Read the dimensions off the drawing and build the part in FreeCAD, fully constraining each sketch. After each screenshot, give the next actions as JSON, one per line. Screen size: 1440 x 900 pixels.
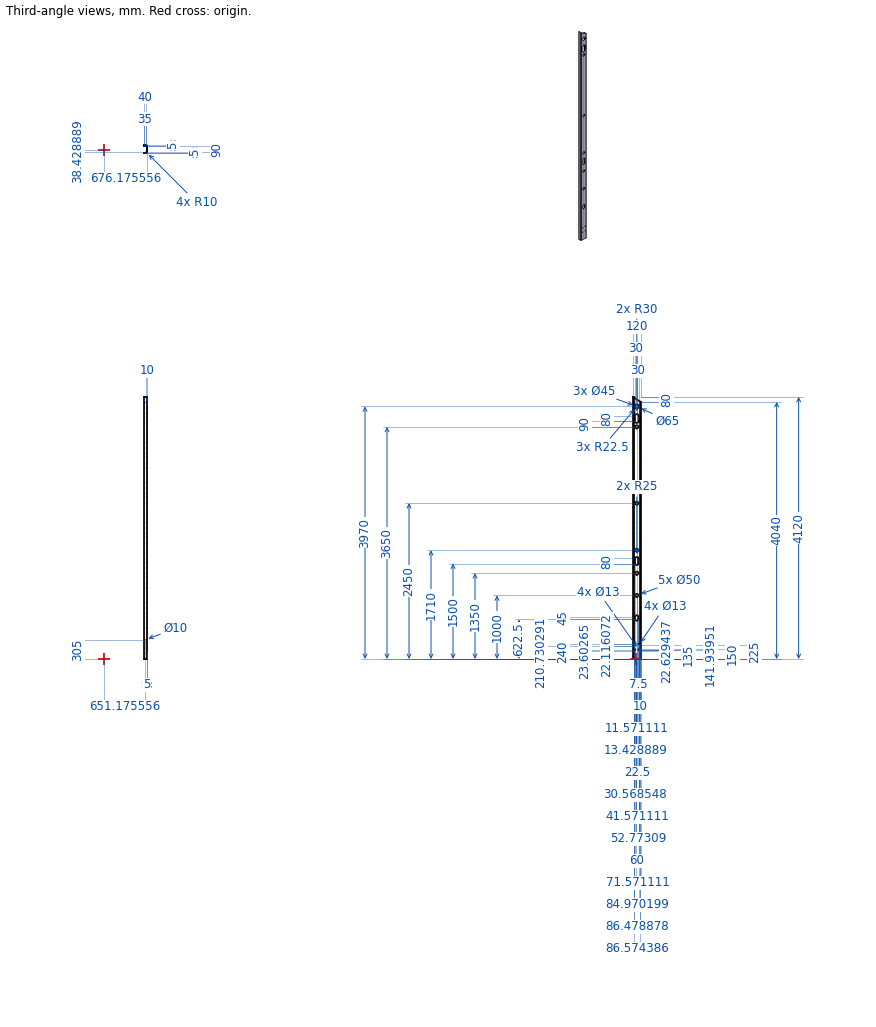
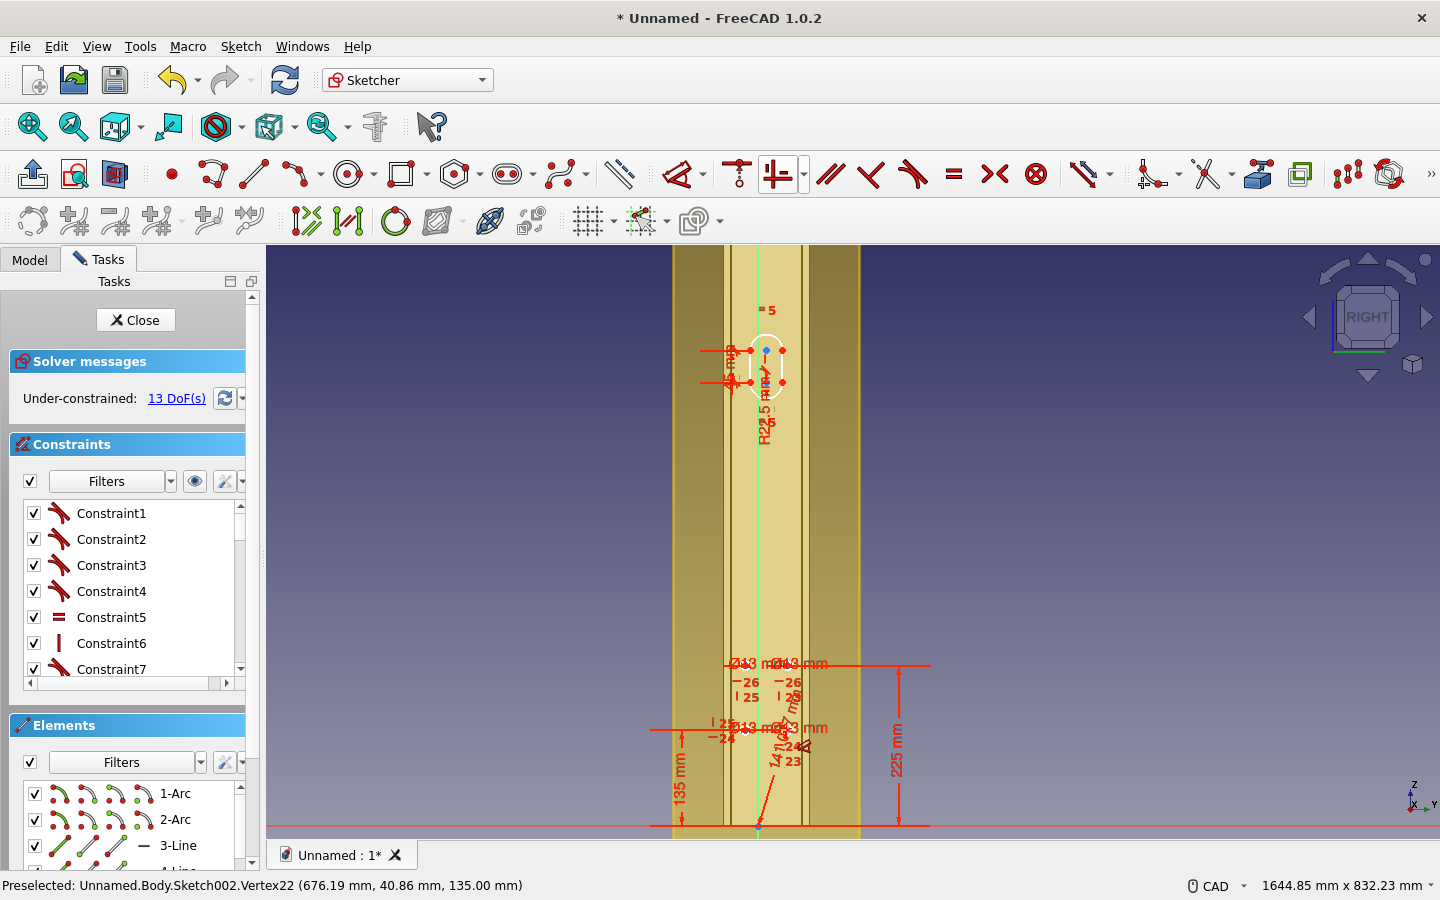
{"action": "left_click", "coordinate": [745, 730]}
{"action": "left_click", "coordinate": [776, 764]}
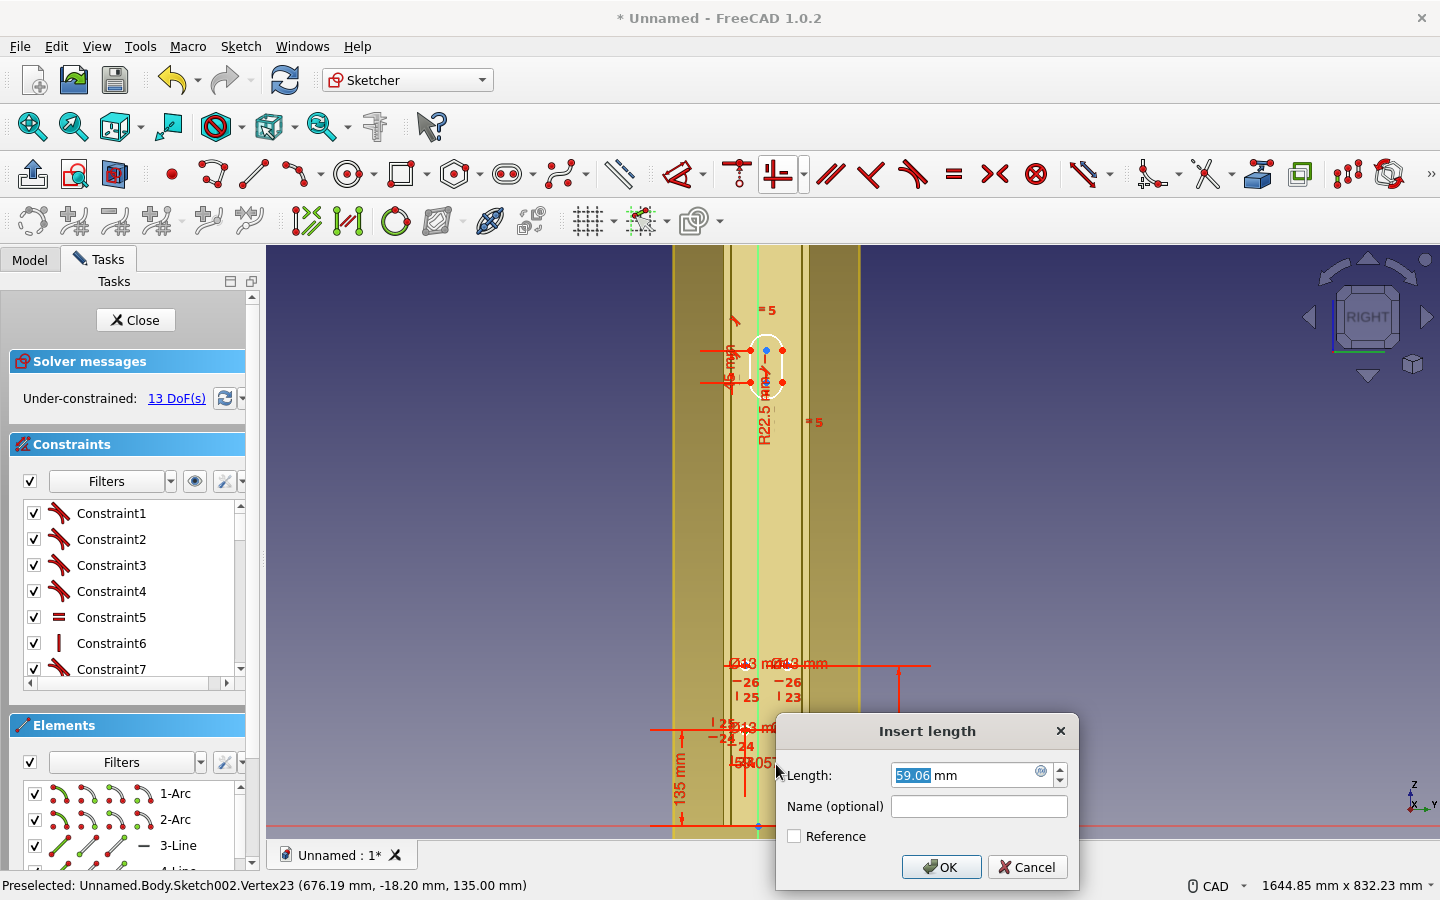
{"action": "type", "text": "60"}
{"action": "key", "text": "Return"}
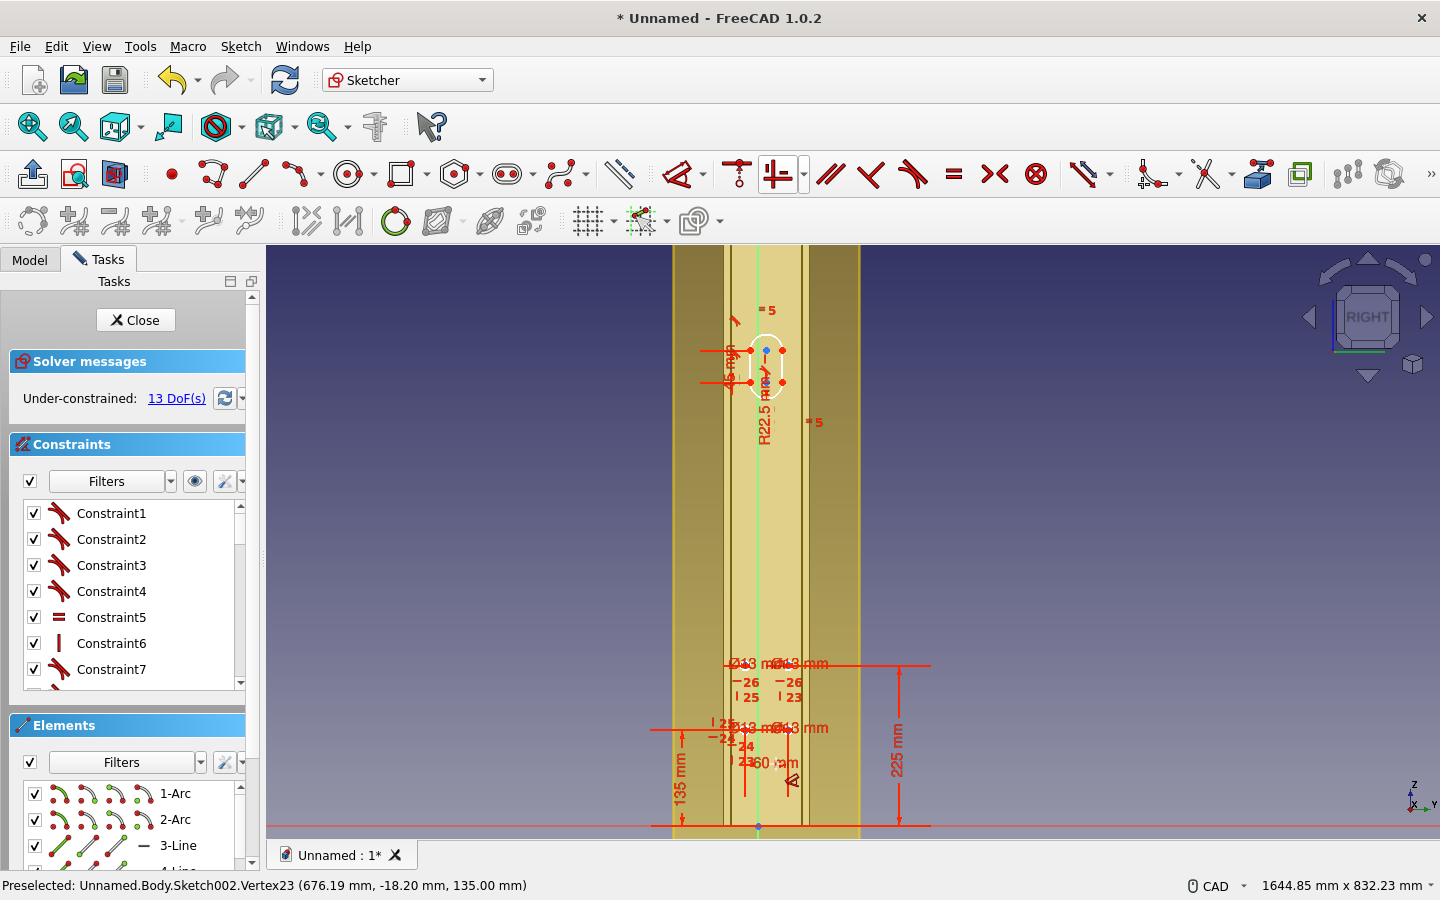
{"action": "scroll", "coordinate": [787, 720], "scroll_direction": "down", "scroll_amount": 10}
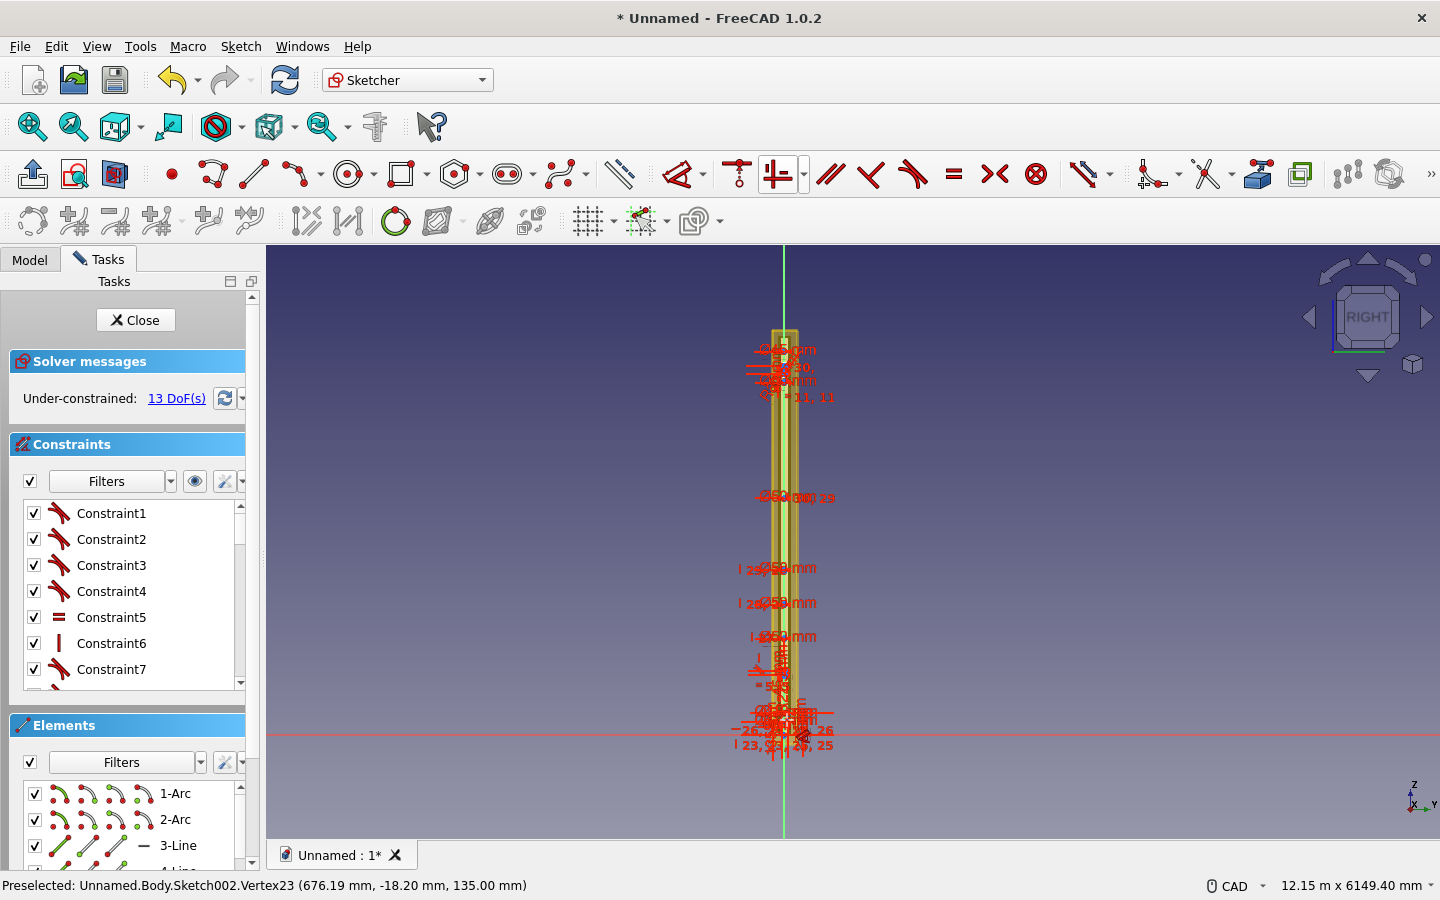
{"action": "scroll", "coordinate": [787, 366], "scroll_direction": "up", "scroll_amount": 14}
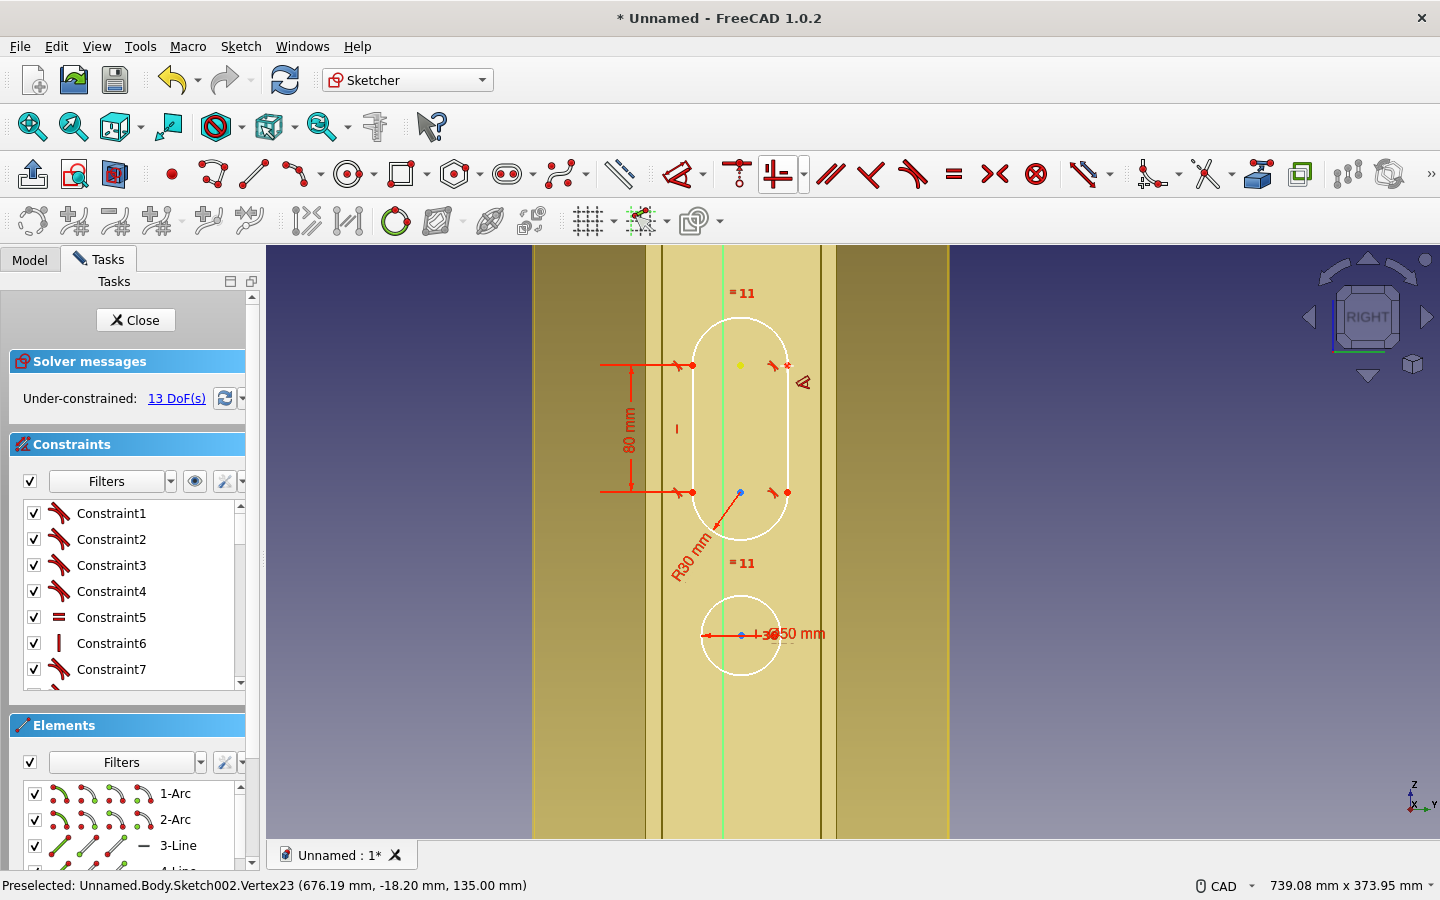
{"action": "left_click", "coordinate": [788, 365]}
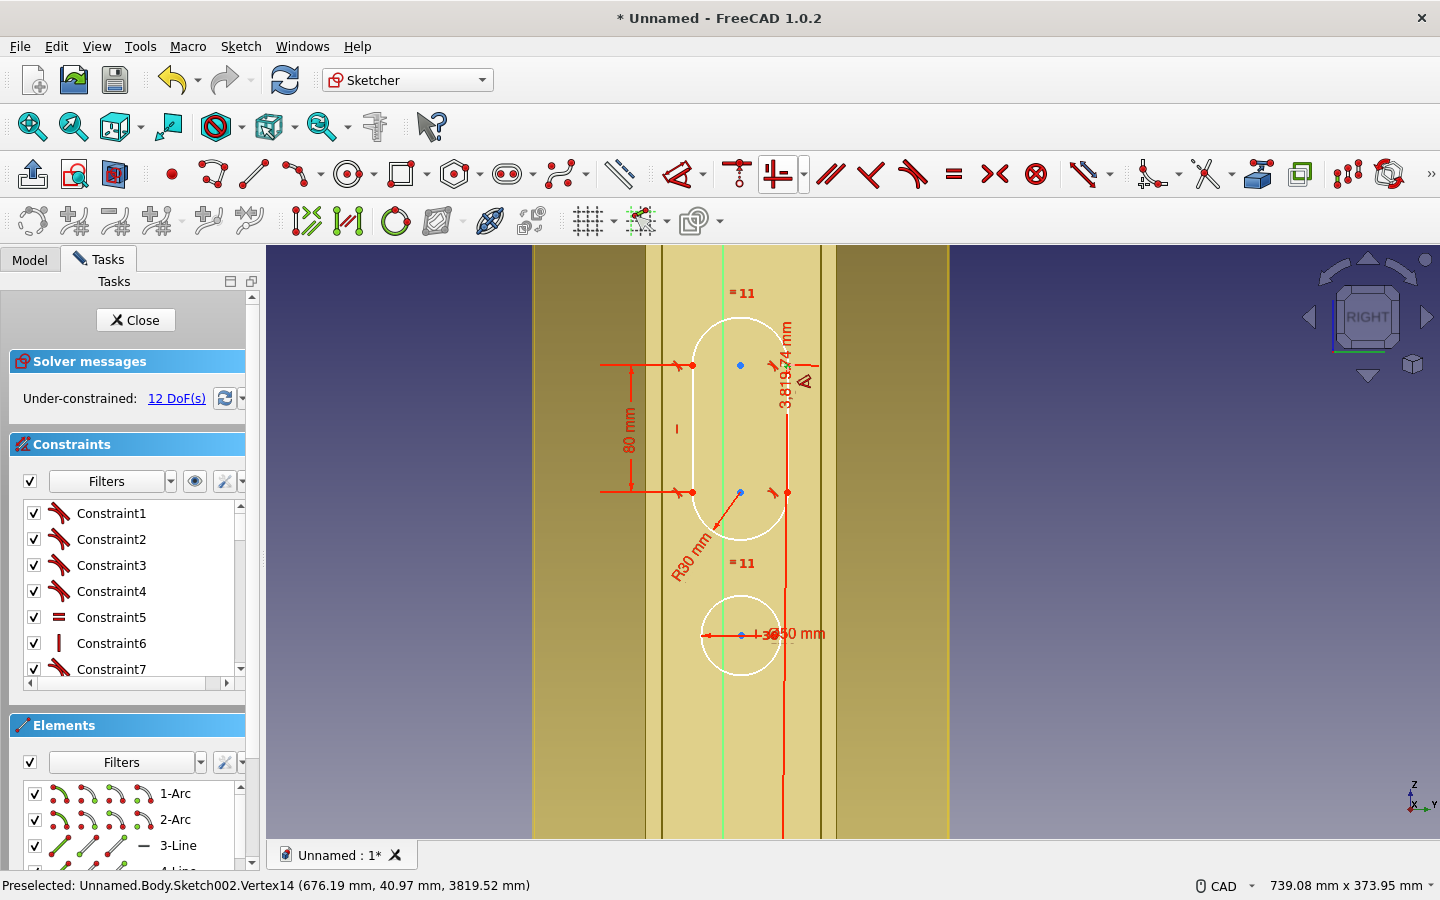
{"action": "scroll", "coordinate": [787, 366], "scroll_direction": "down", "scroll_amount": 14}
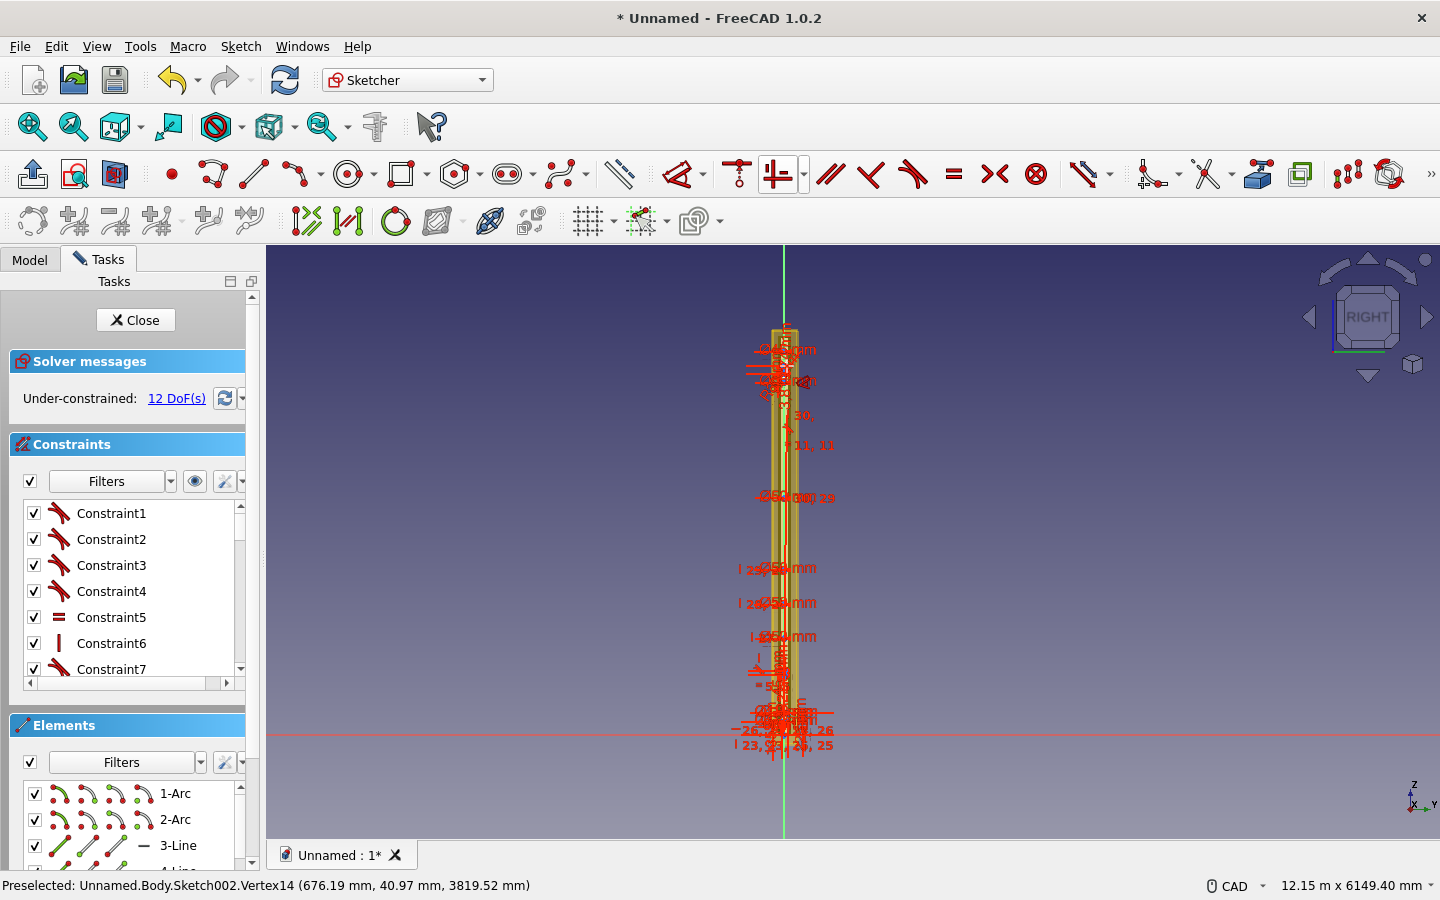
{"action": "scroll", "coordinate": [785, 352], "scroll_direction": "up", "scroll_amount": 14}